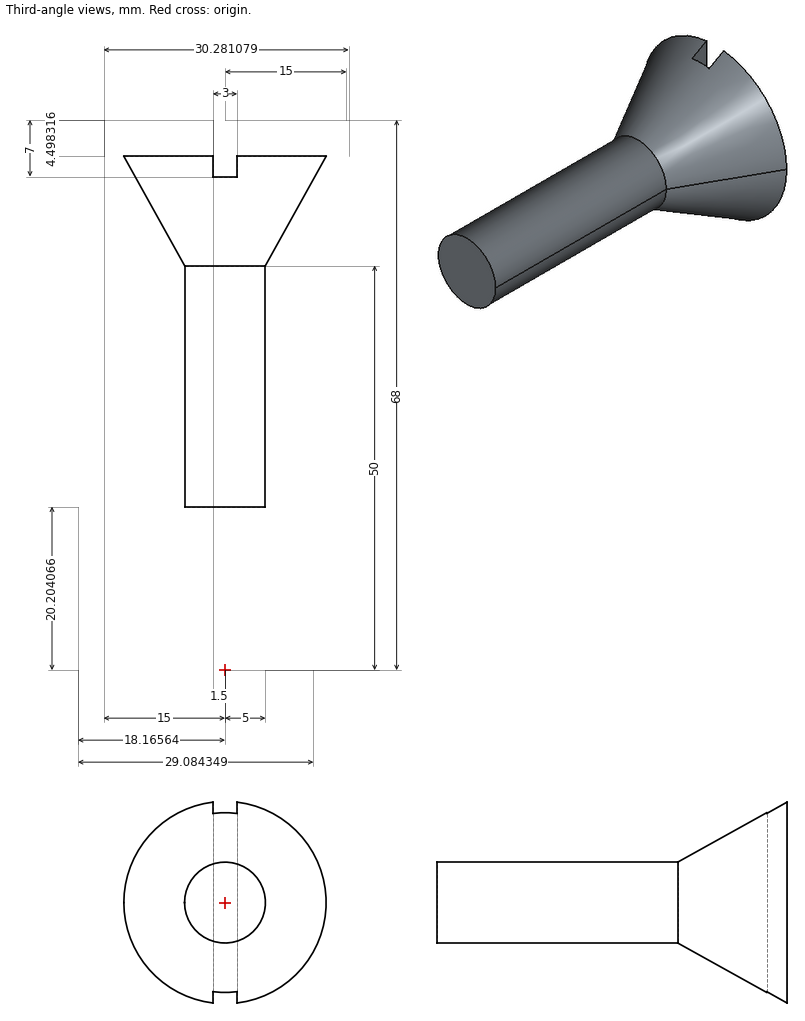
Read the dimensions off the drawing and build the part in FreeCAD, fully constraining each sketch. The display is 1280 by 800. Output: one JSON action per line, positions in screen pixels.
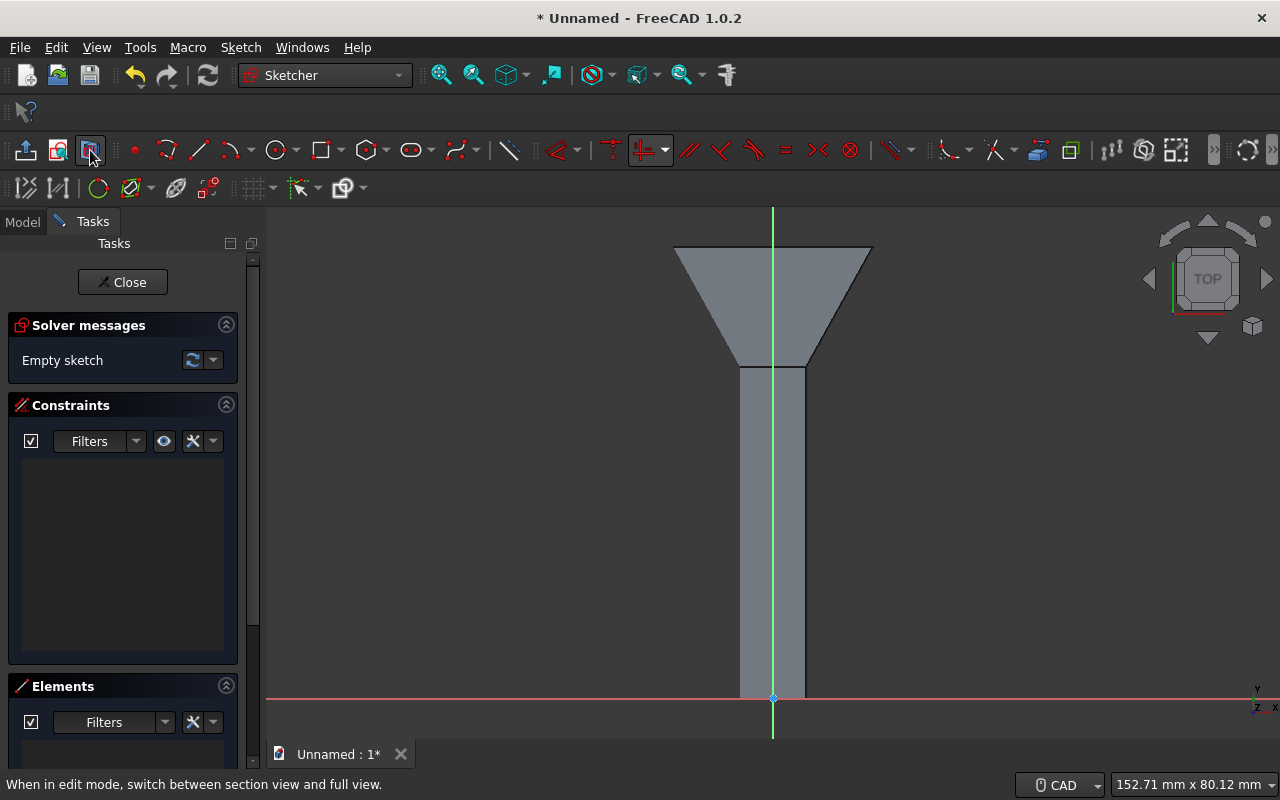
{"action": "scroll", "coordinate": [784, 239], "scroll_direction": "up", "scroll_amount": 10}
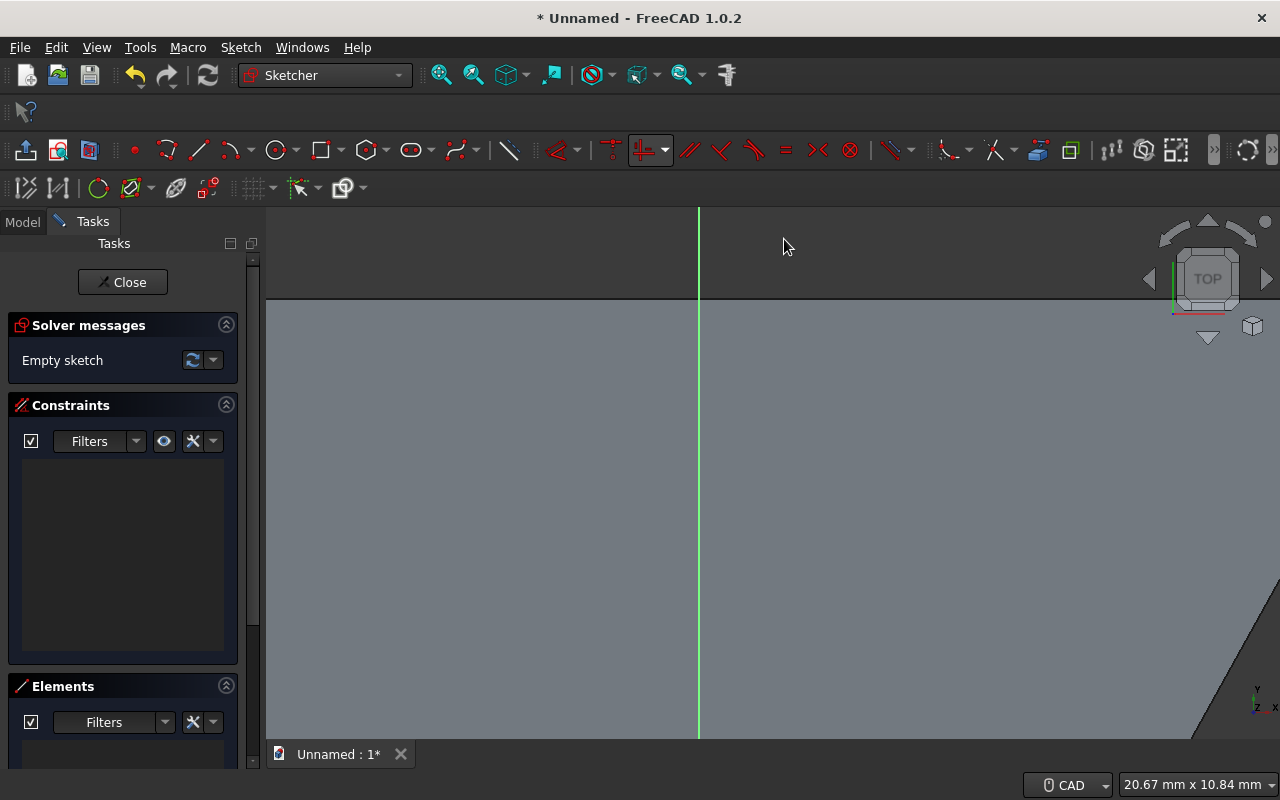
{"action": "key", "text": "g r"}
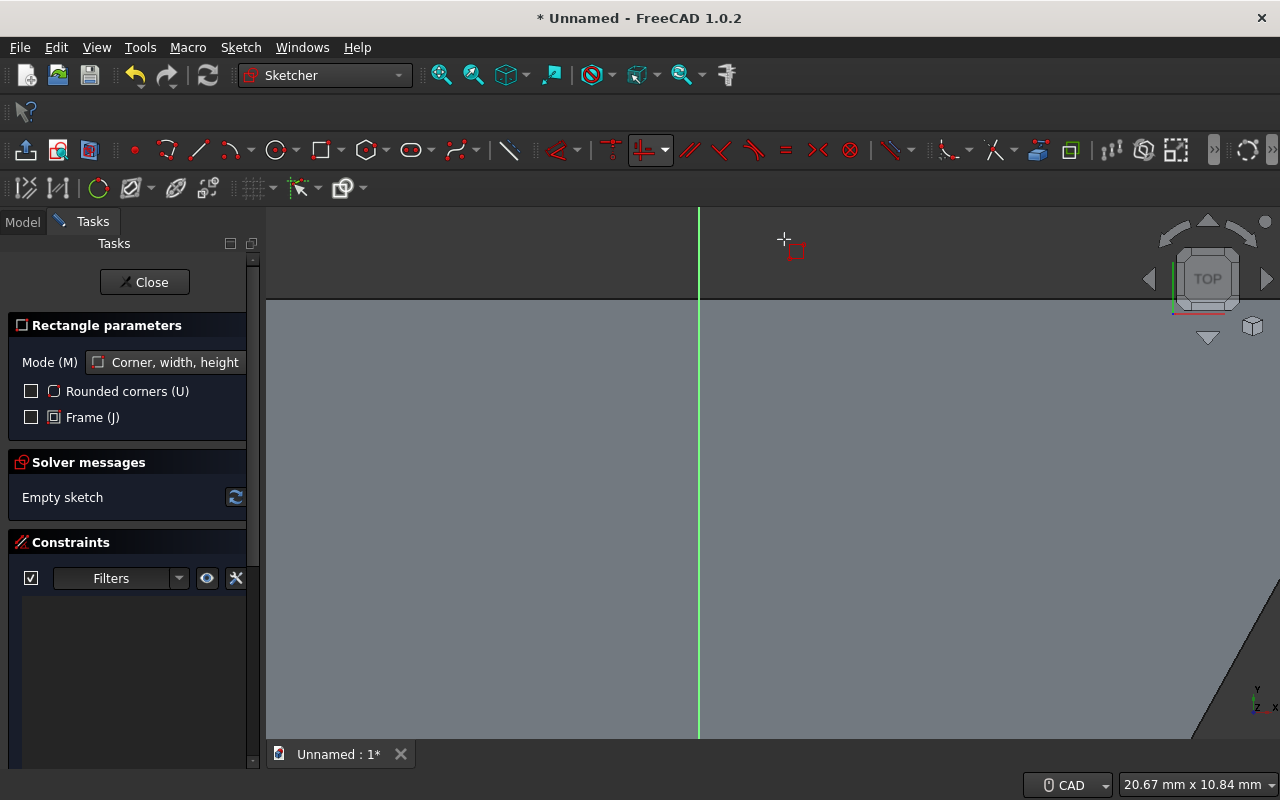
{"action": "left_click", "coordinate": [626, 299]}
{"action": "left_click", "coordinate": [773, 643]}
{"action": "key", "text": "Escape"}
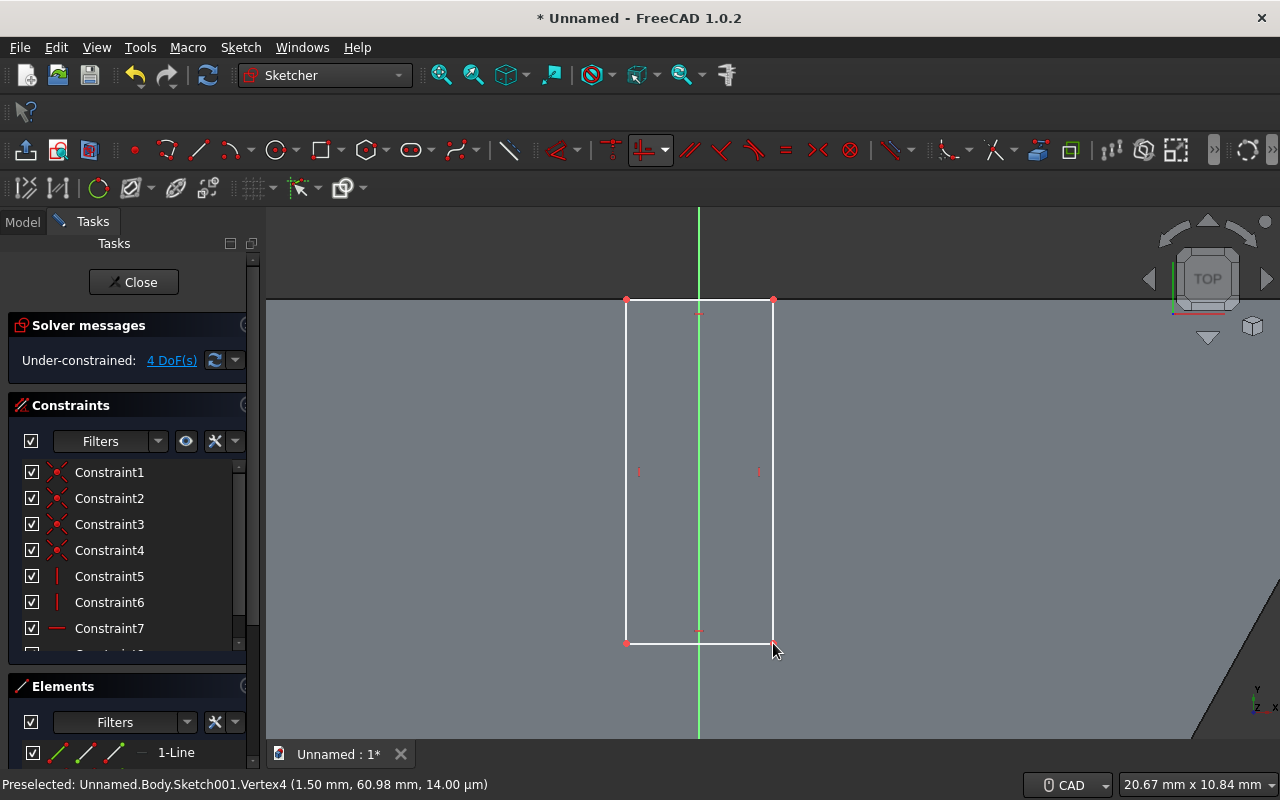
{"action": "key", "text": "d"}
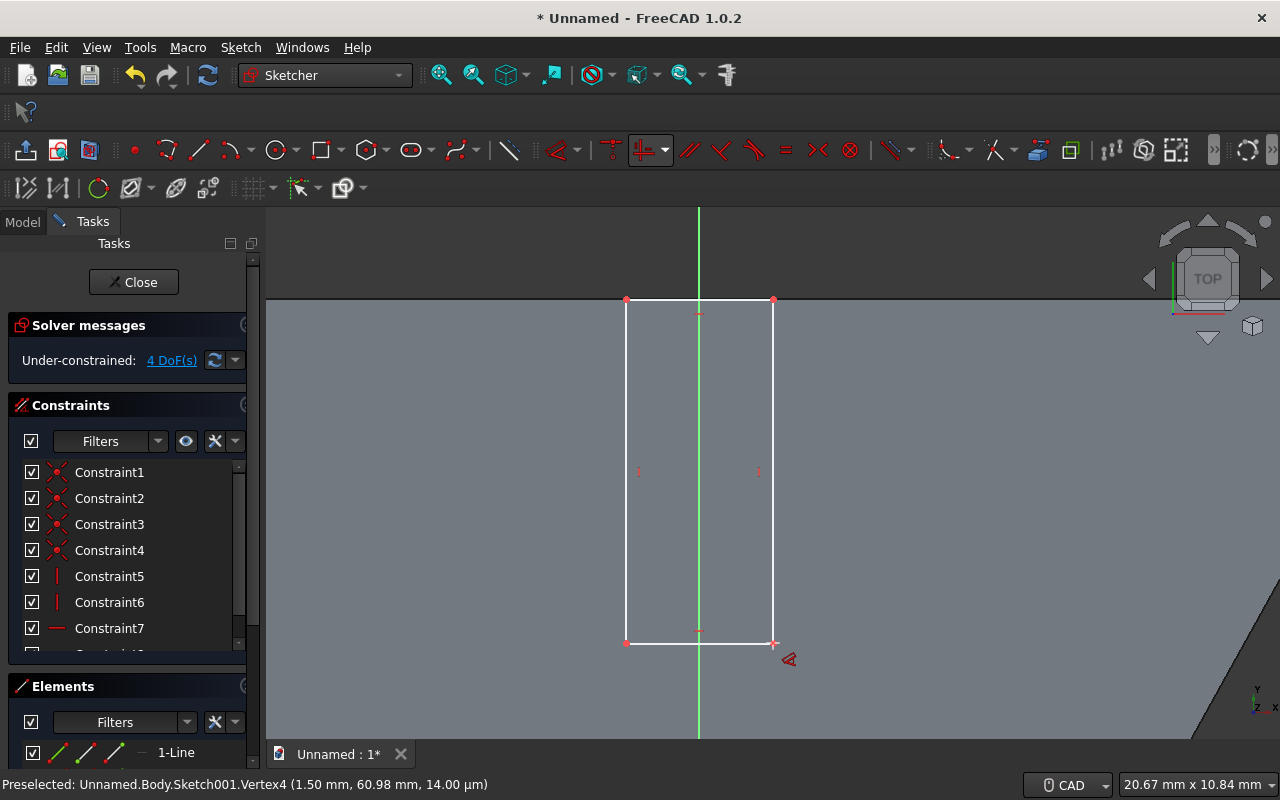
{"action": "left_click", "coordinate": [626, 403]}
{"action": "left_click", "coordinate": [592, 472]}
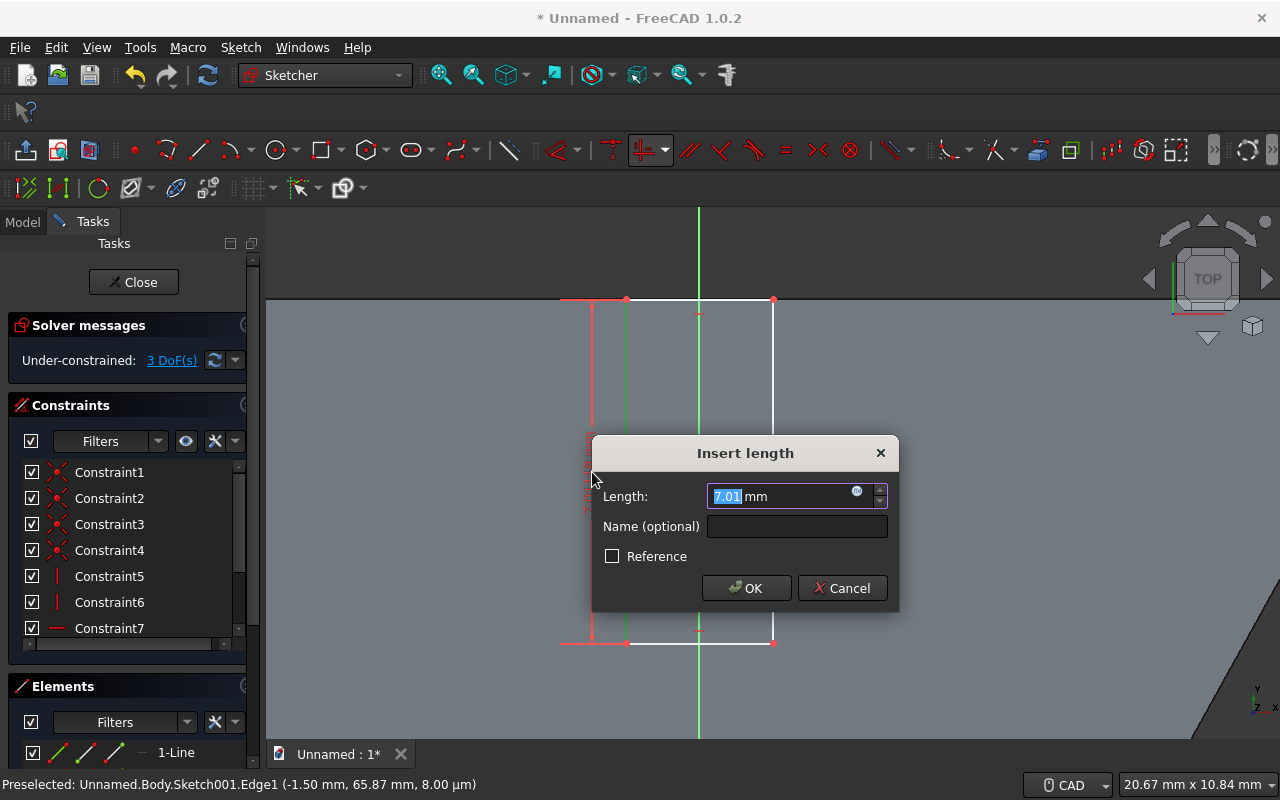
{"action": "type", "text": "7"}
{"action": "key", "text": "Return"}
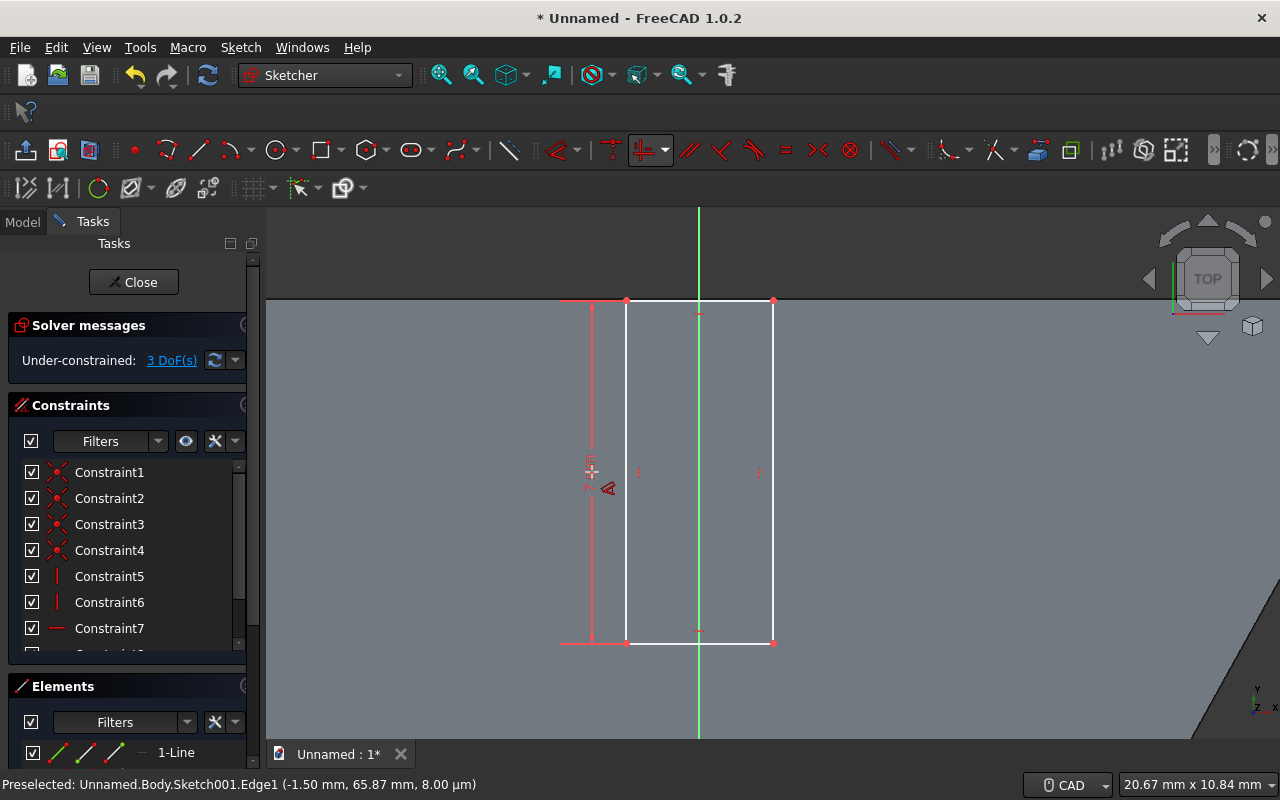
{"action": "left_click", "coordinate": [670, 644]}
{"action": "left_click", "coordinate": [666, 678]}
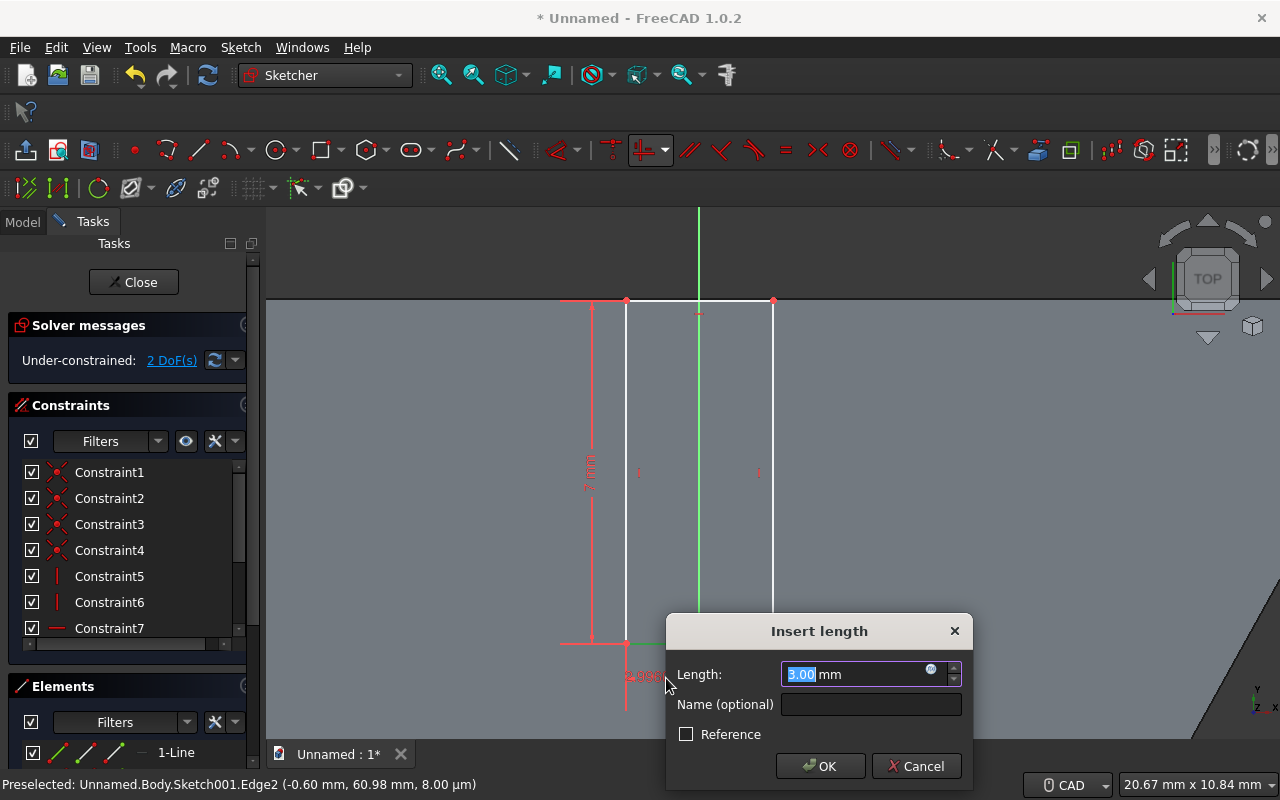
{"action": "type", "text": "3"}
{"action": "key", "text": "Return"}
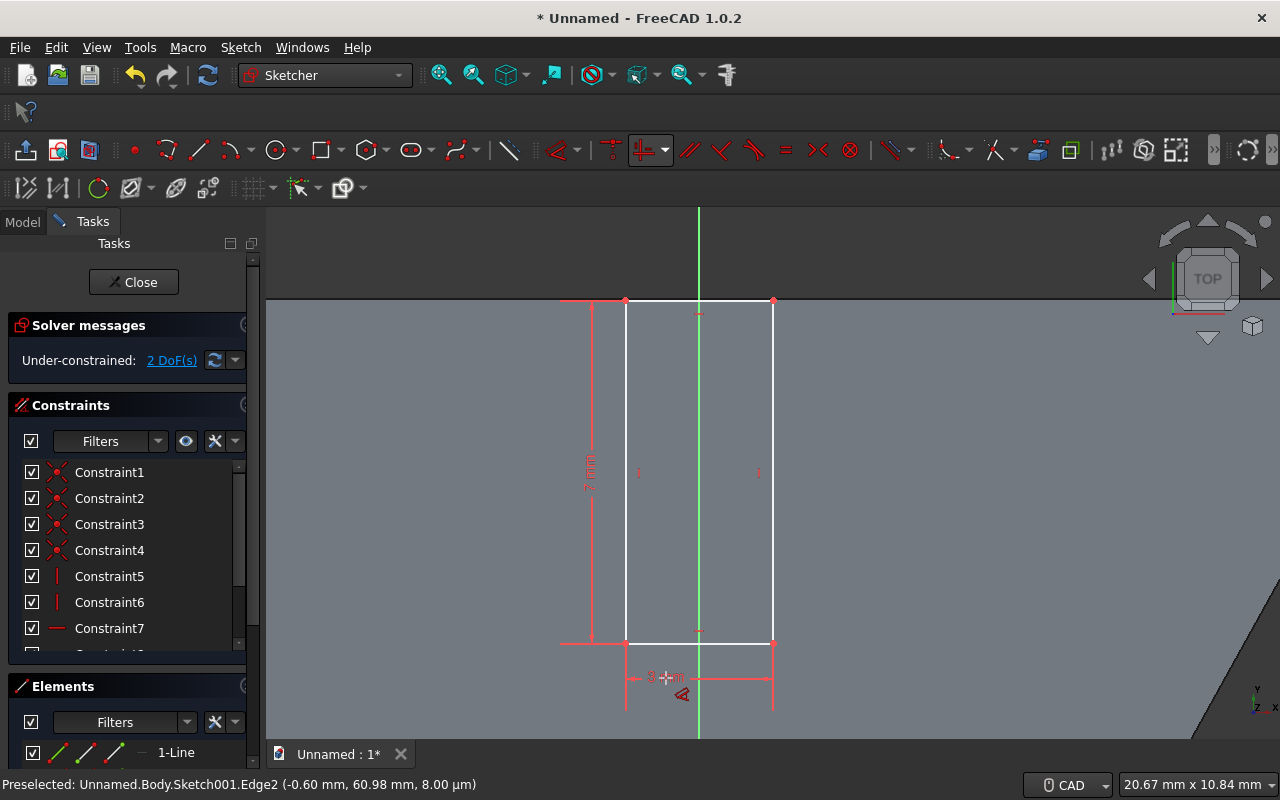
{"action": "left_click", "coordinate": [626, 301]}
{"action": "left_click", "coordinate": [592, 506]}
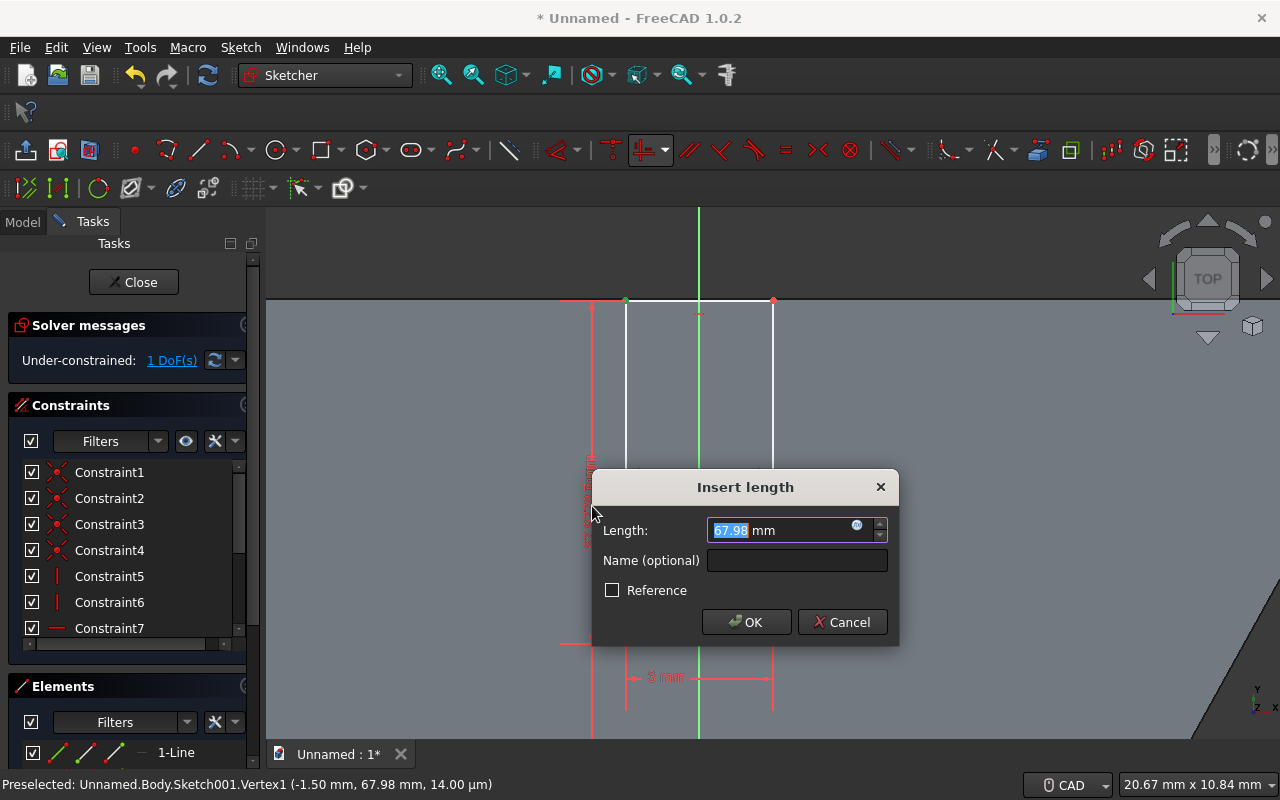
{"action": "type", "text": "68"}
{"action": "key", "text": "Return"}